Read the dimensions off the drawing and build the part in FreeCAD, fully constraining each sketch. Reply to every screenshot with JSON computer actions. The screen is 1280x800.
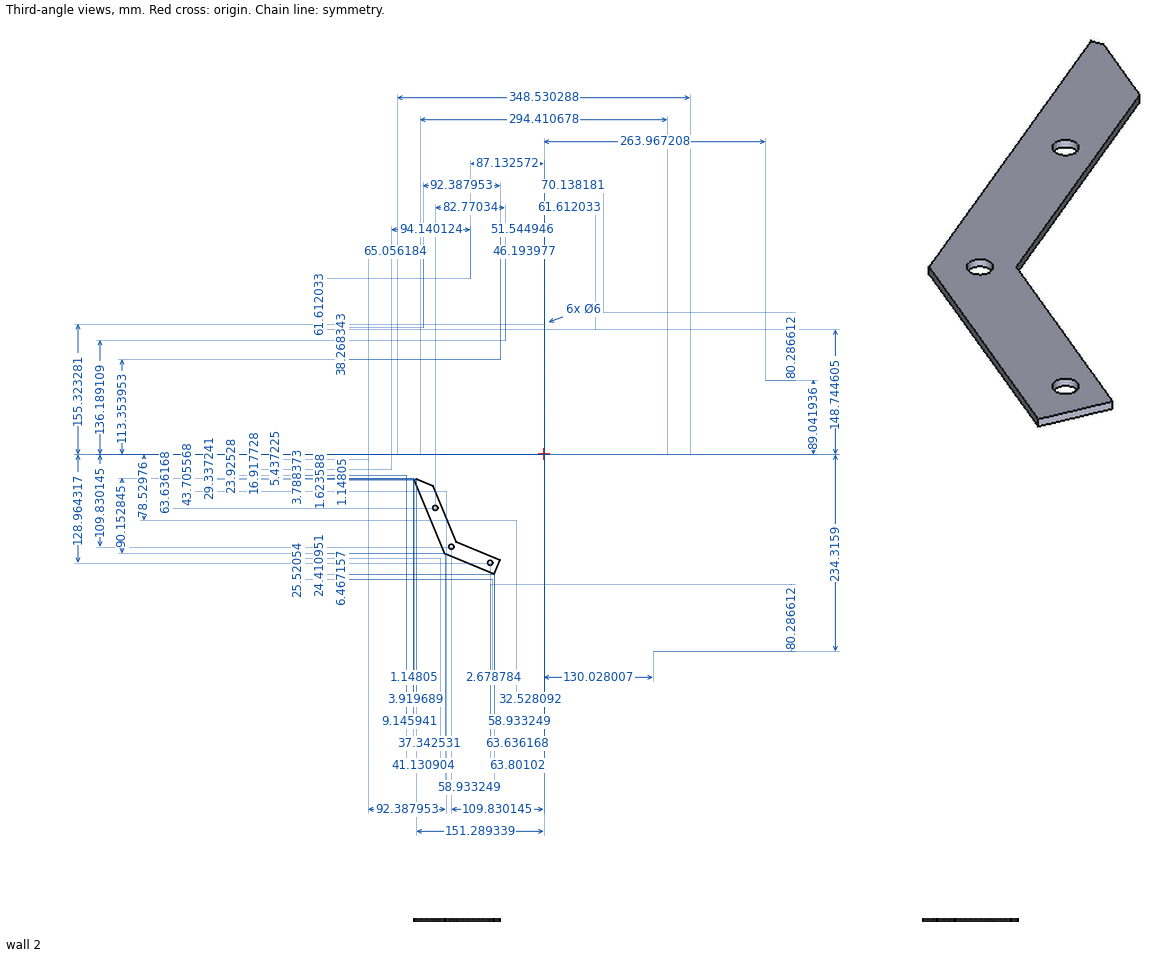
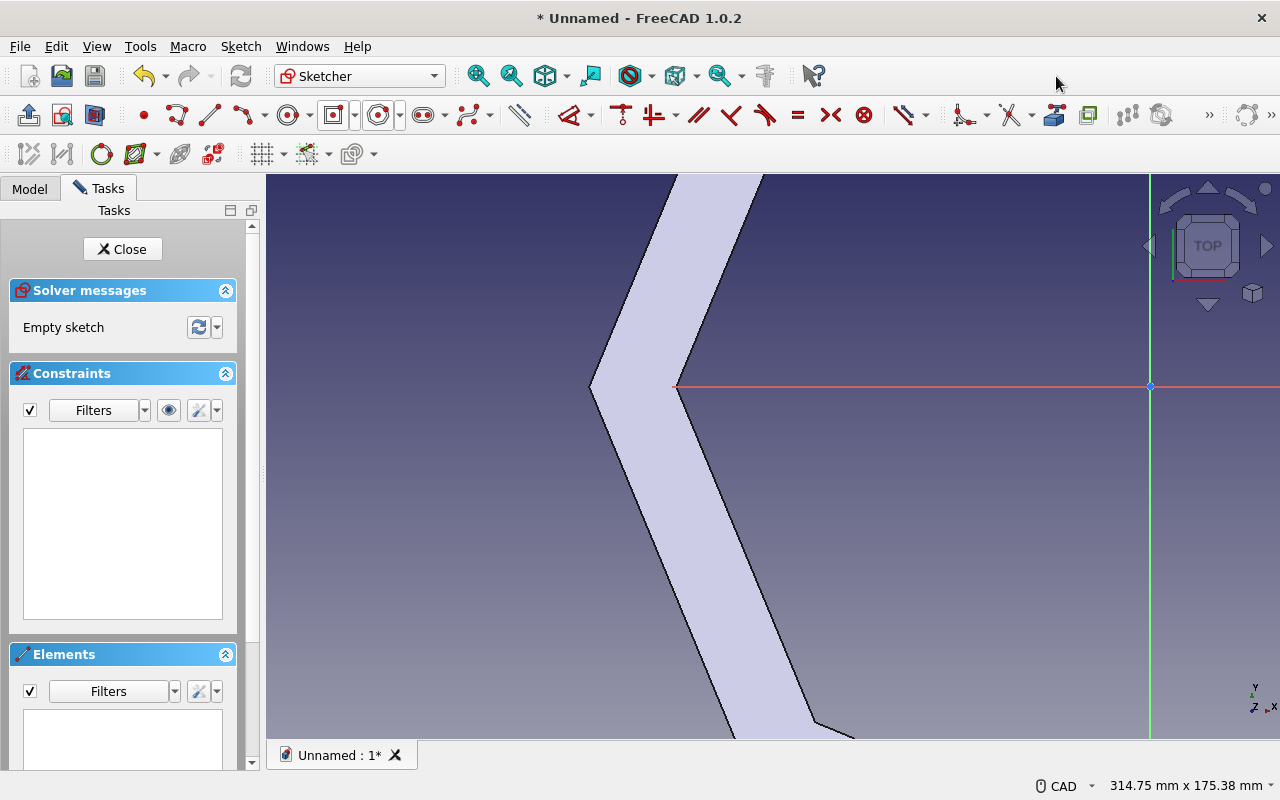
{"action": "scroll", "coordinate": [373, 441], "scroll_direction": "down", "scroll_amount": 6}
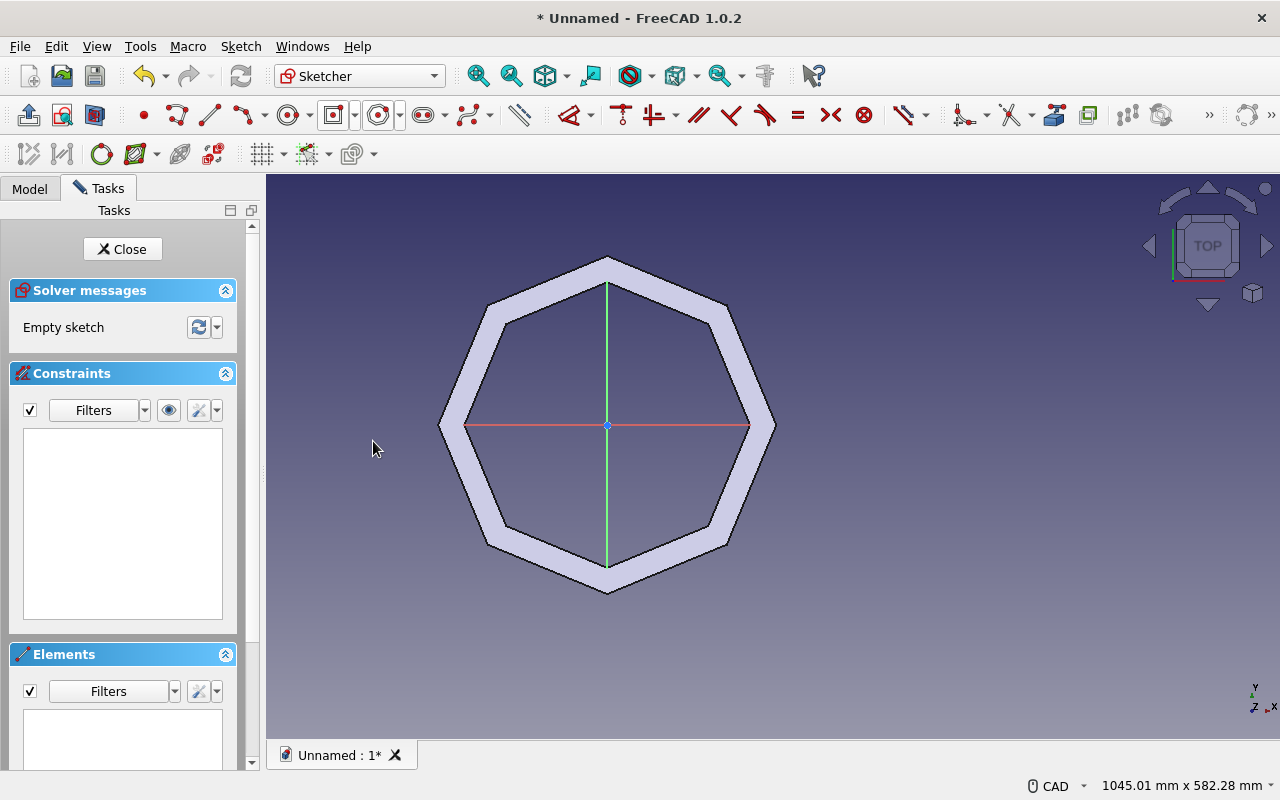
{"action": "left_click", "coordinate": [177, 116]}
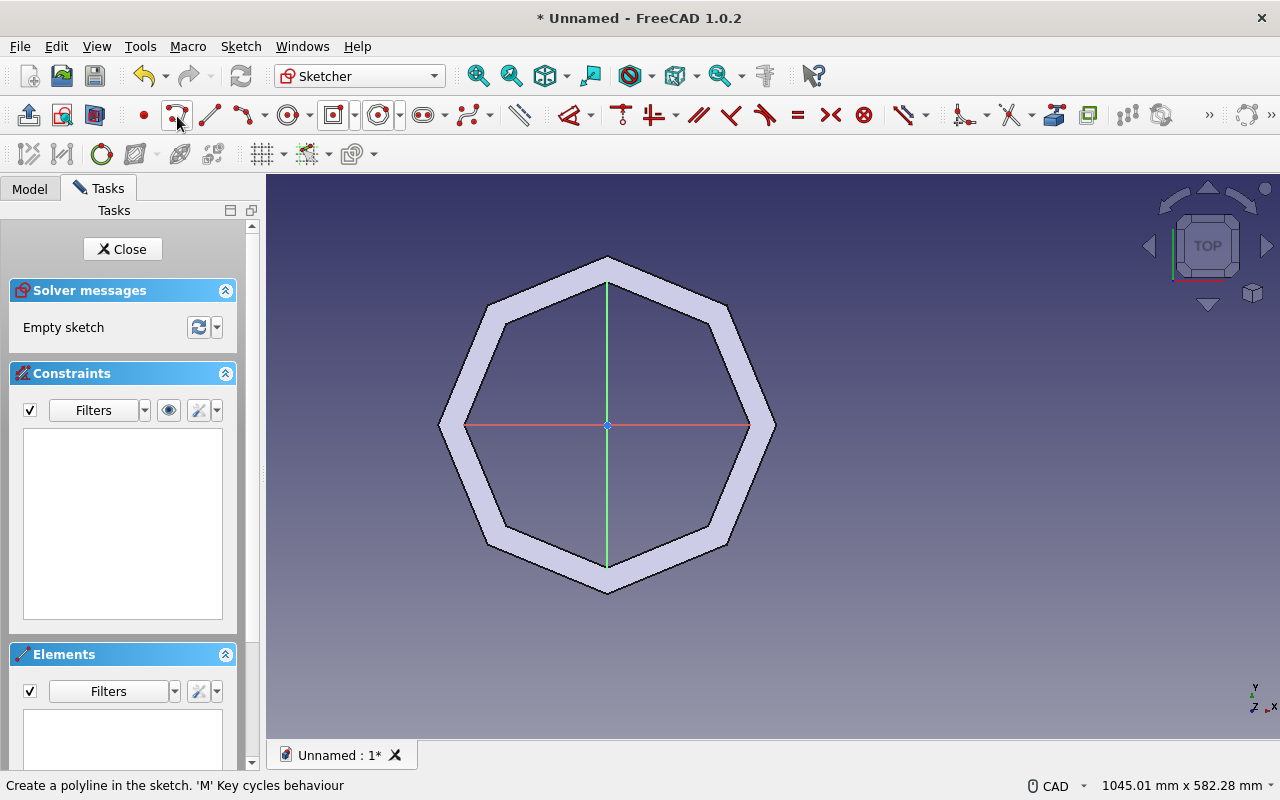
{"action": "left_click", "coordinate": [545, 575]}
{"action": "left_click", "coordinate": [733, 652]}
{"action": "left_click", "coordinate": [863, 339]}
{"action": "left_click", "coordinate": [675, 261]}
{"action": "left_click", "coordinate": [545, 576]}
{"action": "key", "text": "Escape"}
{"action": "key", "text": "Escape"}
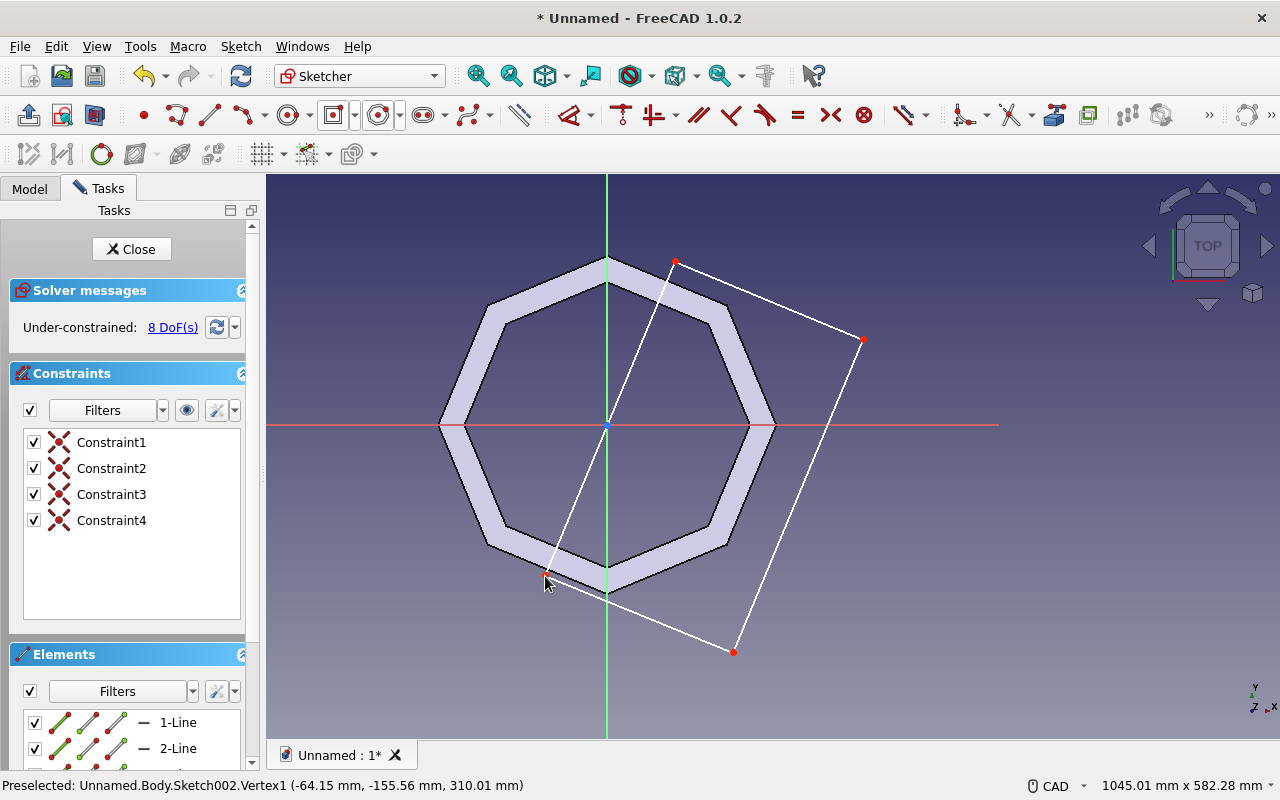
{"action": "left_click", "coordinate": [568, 116]}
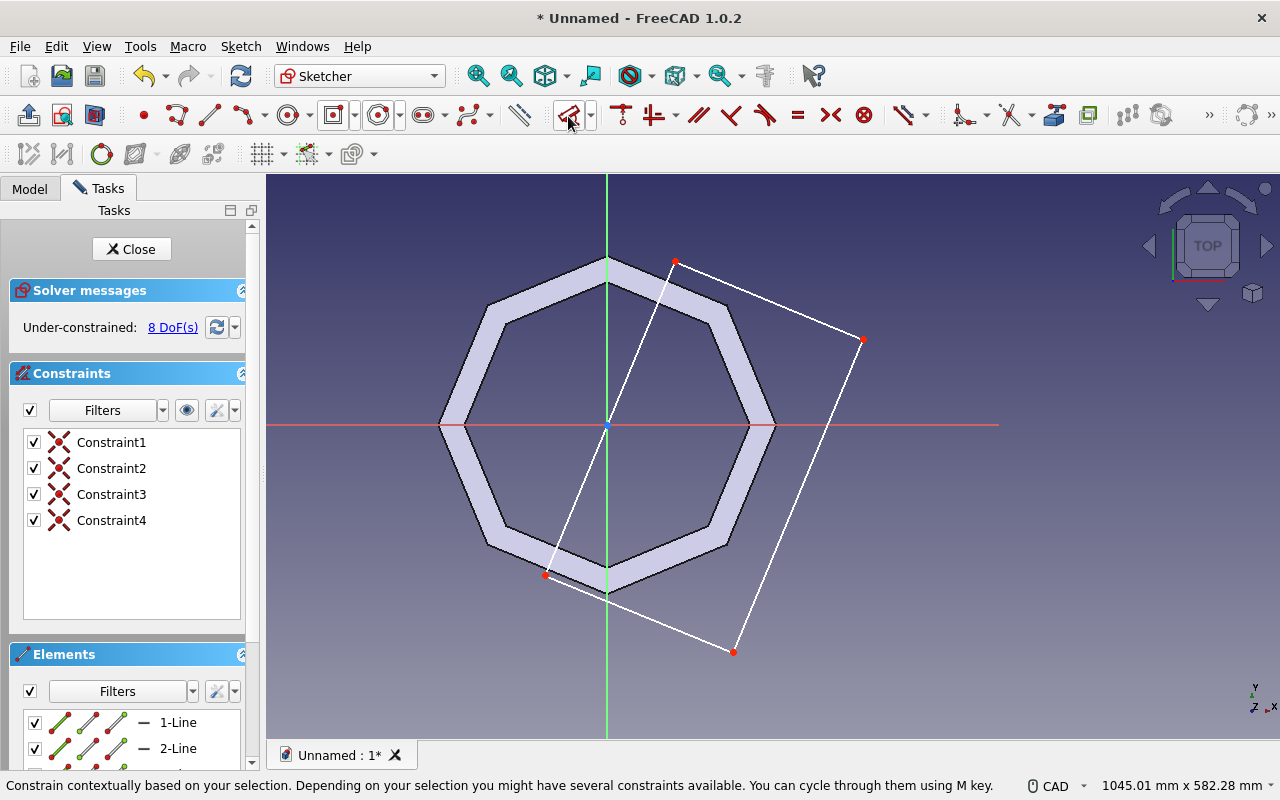
{"action": "left_click", "coordinate": [545, 576]}
{"action": "left_click", "coordinate": [576, 610]}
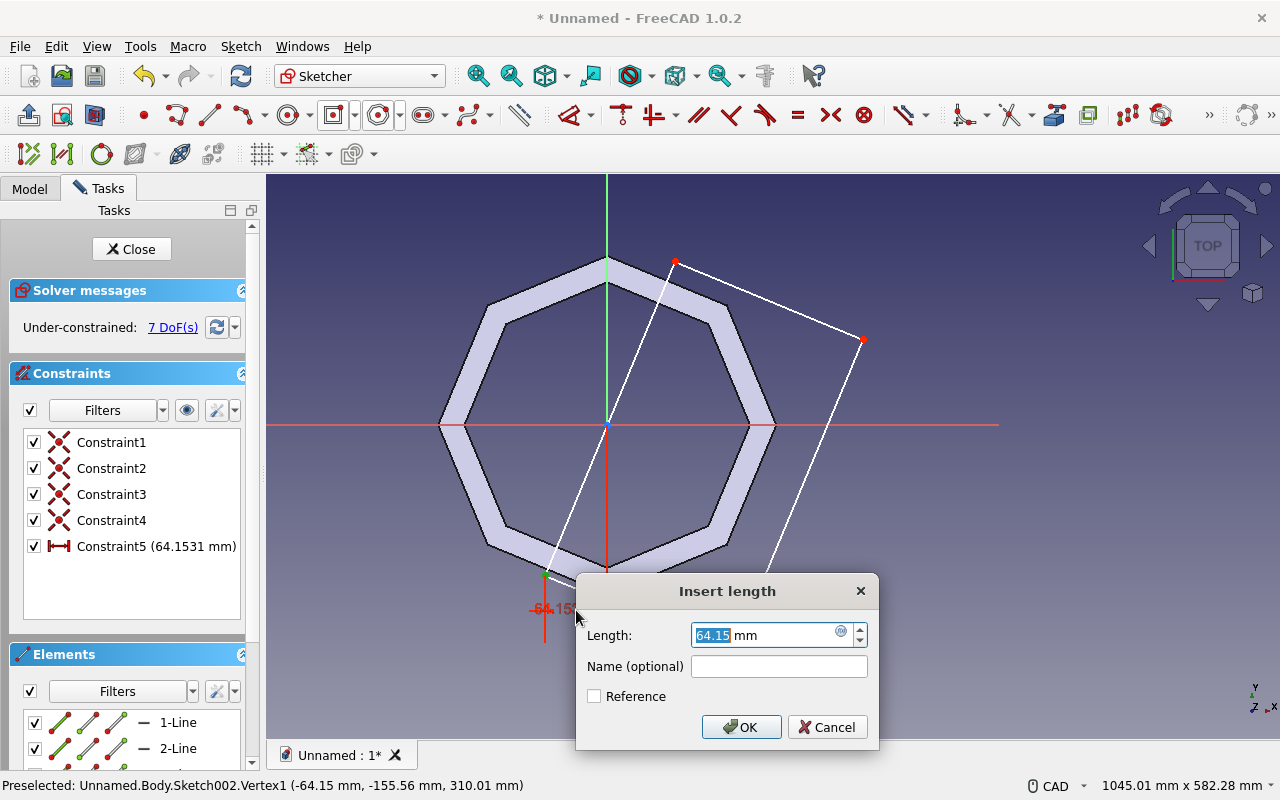
{"action": "type", "text": "63.80102"}
{"action": "key", "text": "Return"}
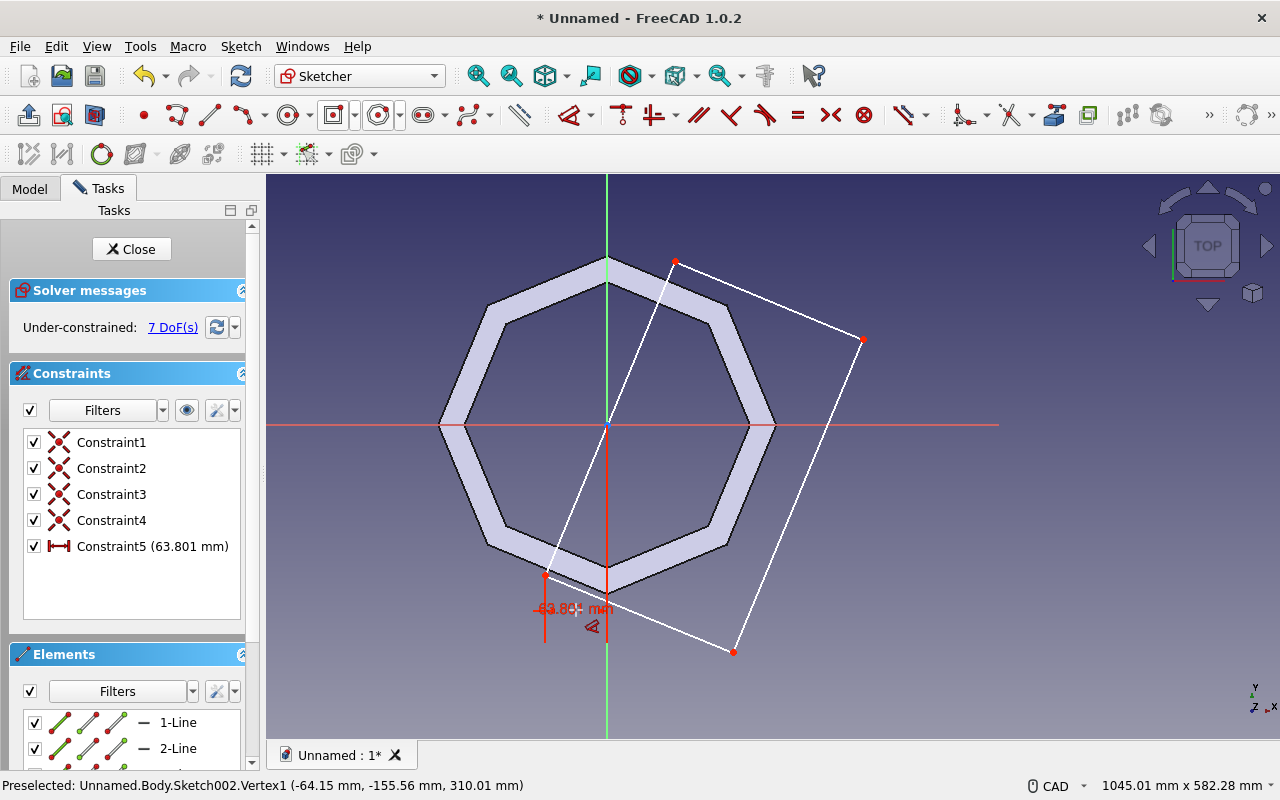
{"action": "left_click", "coordinate": [733, 653]}
{"action": "left_click", "coordinate": [573, 459]}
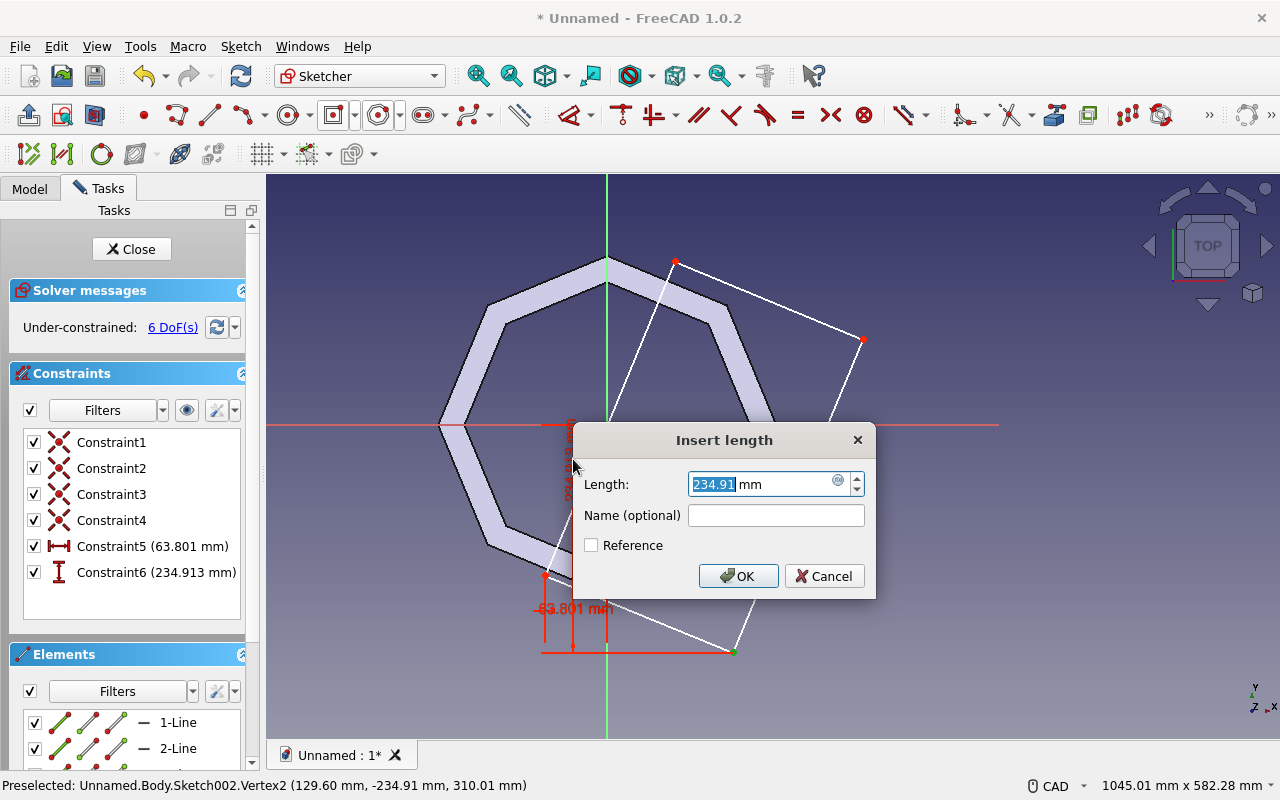
{"action": "type", "text": "234.3159"}
{"action": "key", "text": "Return"}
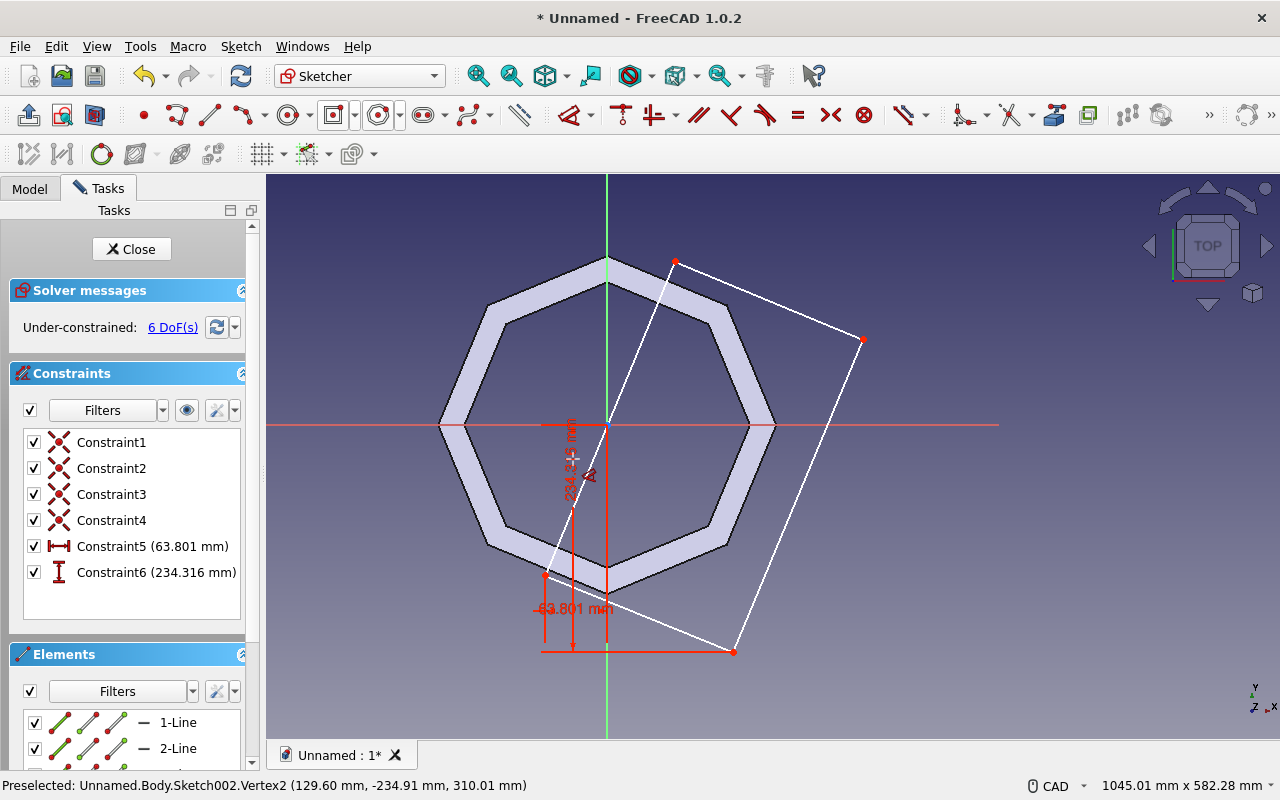
{"action": "left_click", "coordinate": [863, 340]}
{"action": "left_click", "coordinate": [897, 383]}